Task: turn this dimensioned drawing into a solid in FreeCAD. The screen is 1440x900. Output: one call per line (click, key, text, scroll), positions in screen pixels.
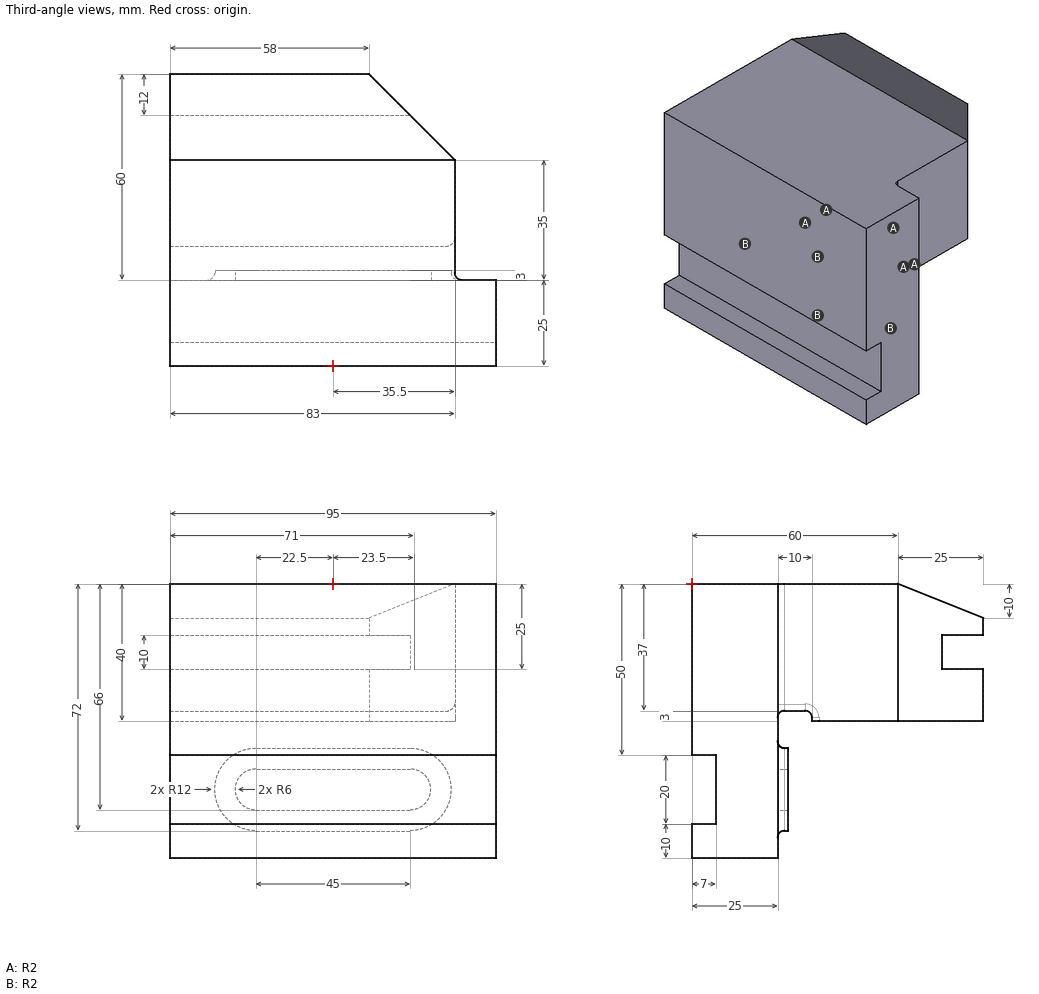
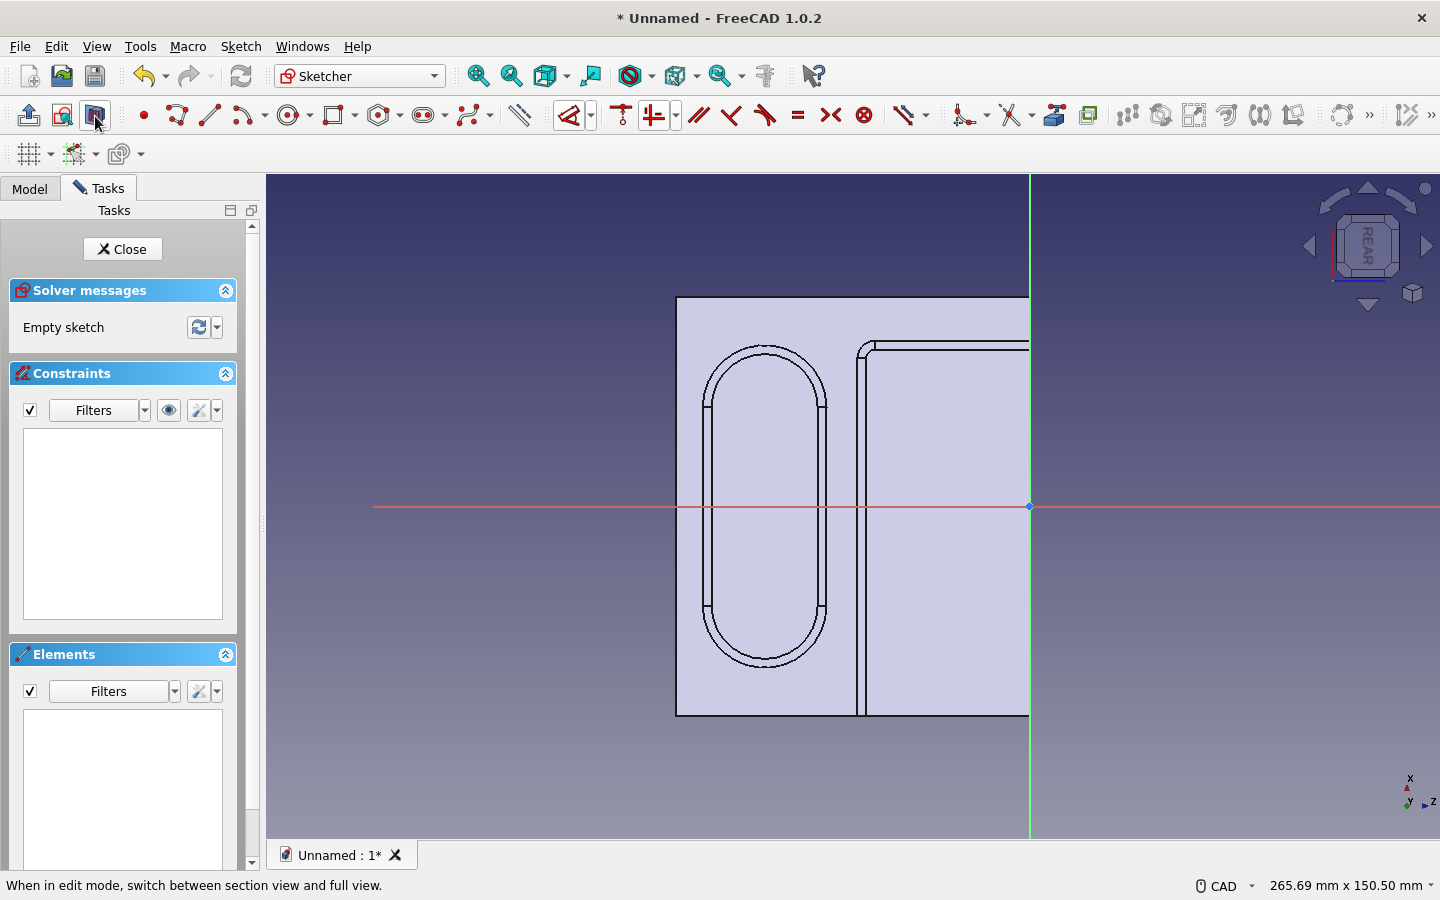
scroll(1005, 507, up, 3)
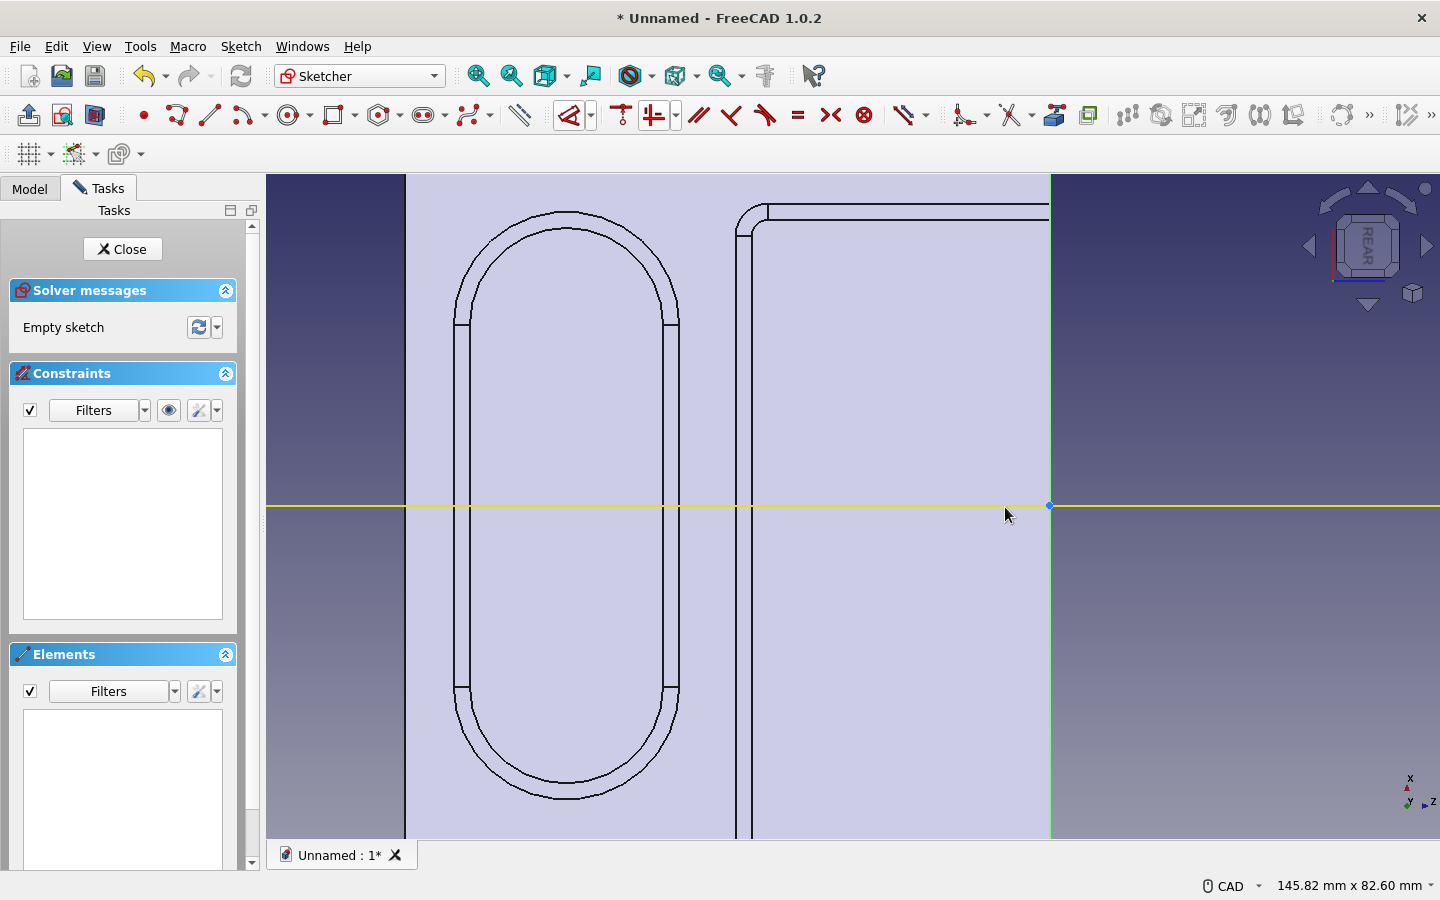
click(422, 116)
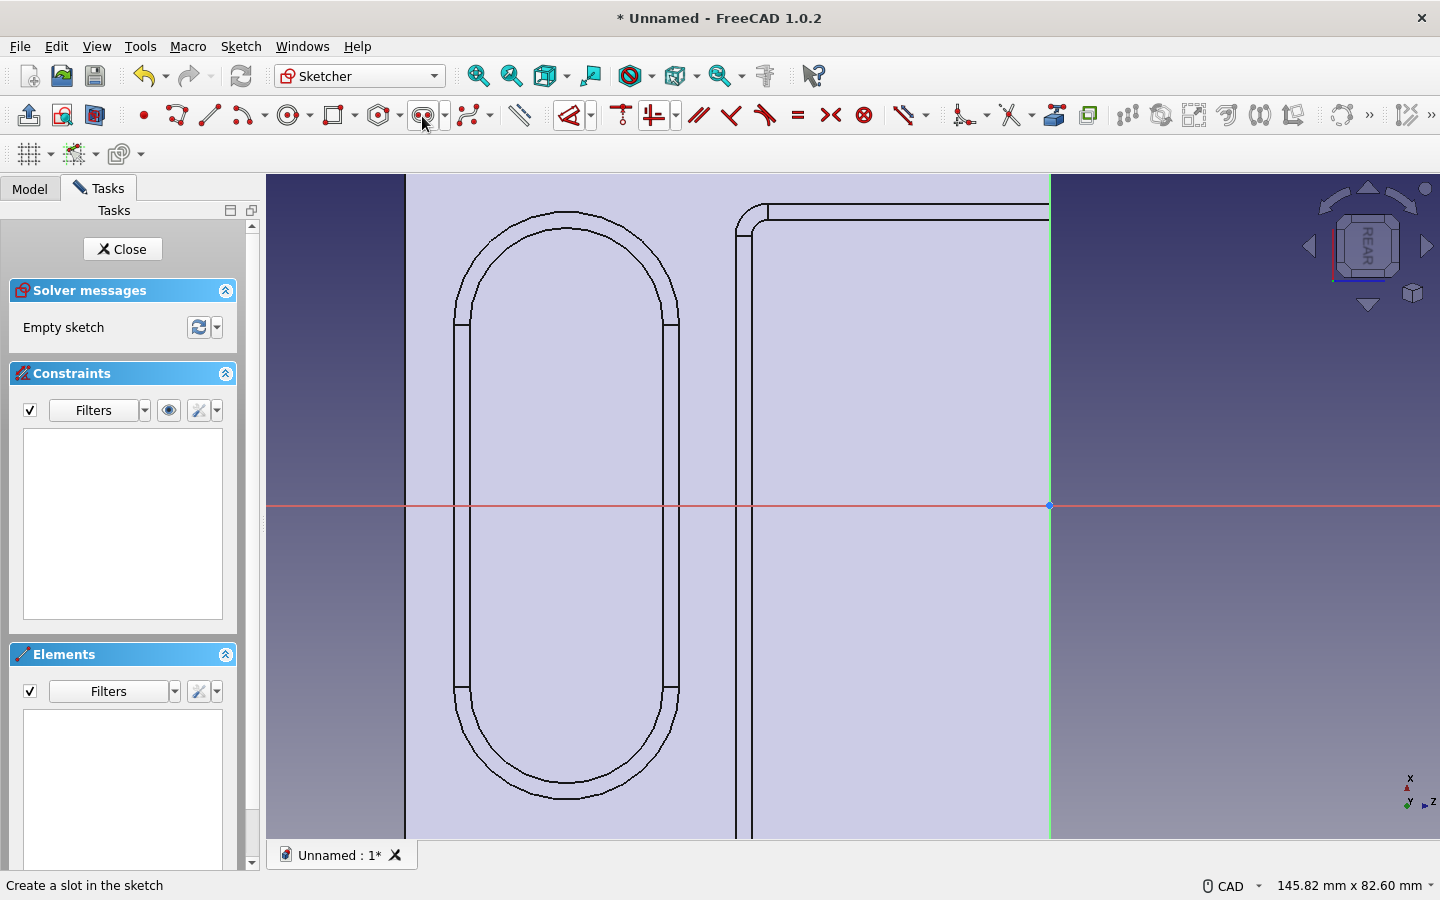
click(566, 687)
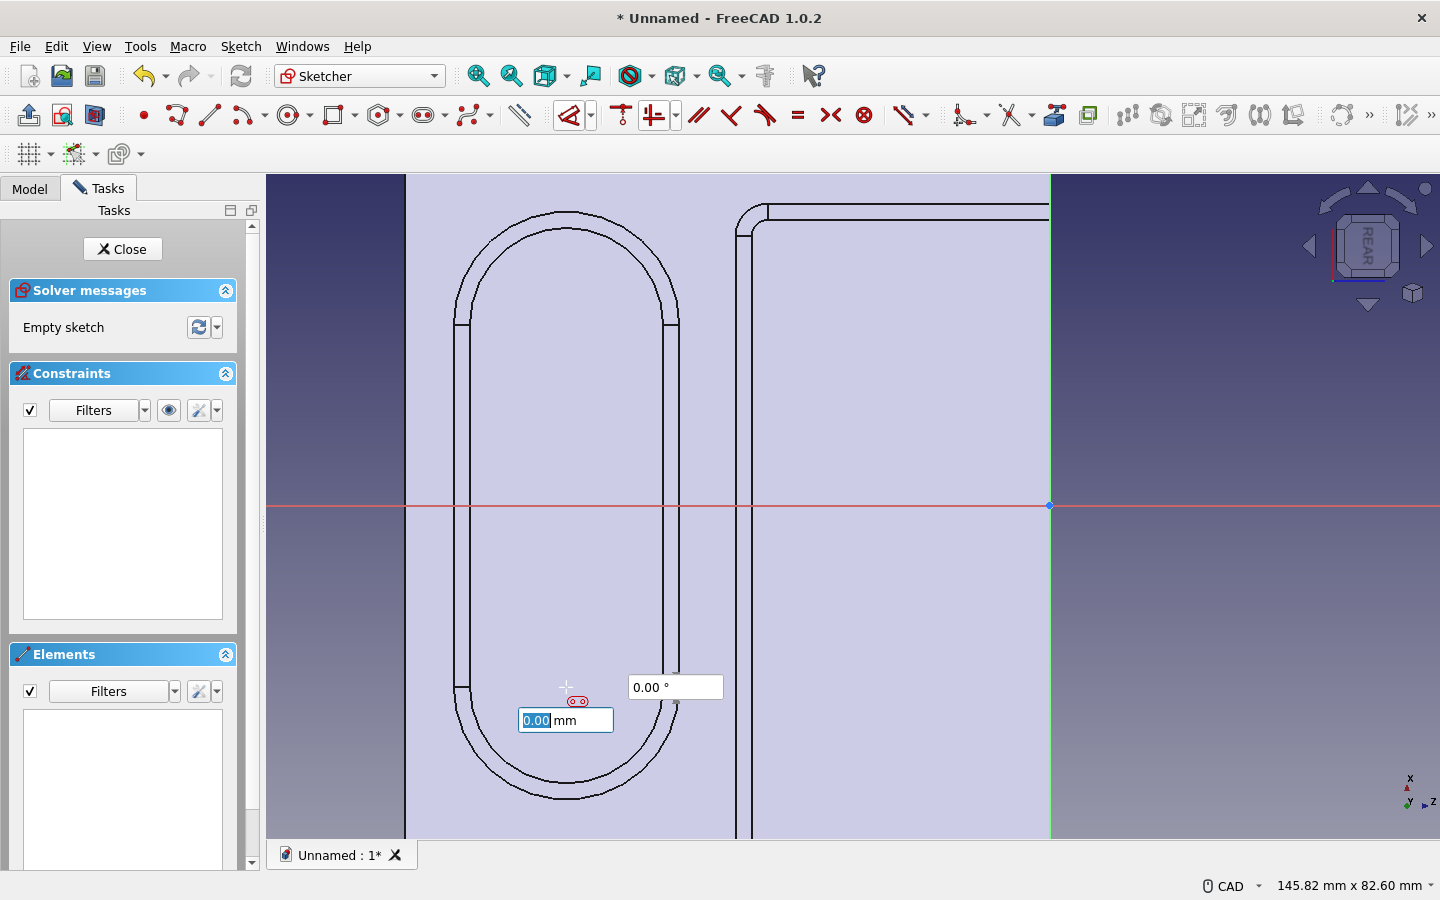
click(566, 325)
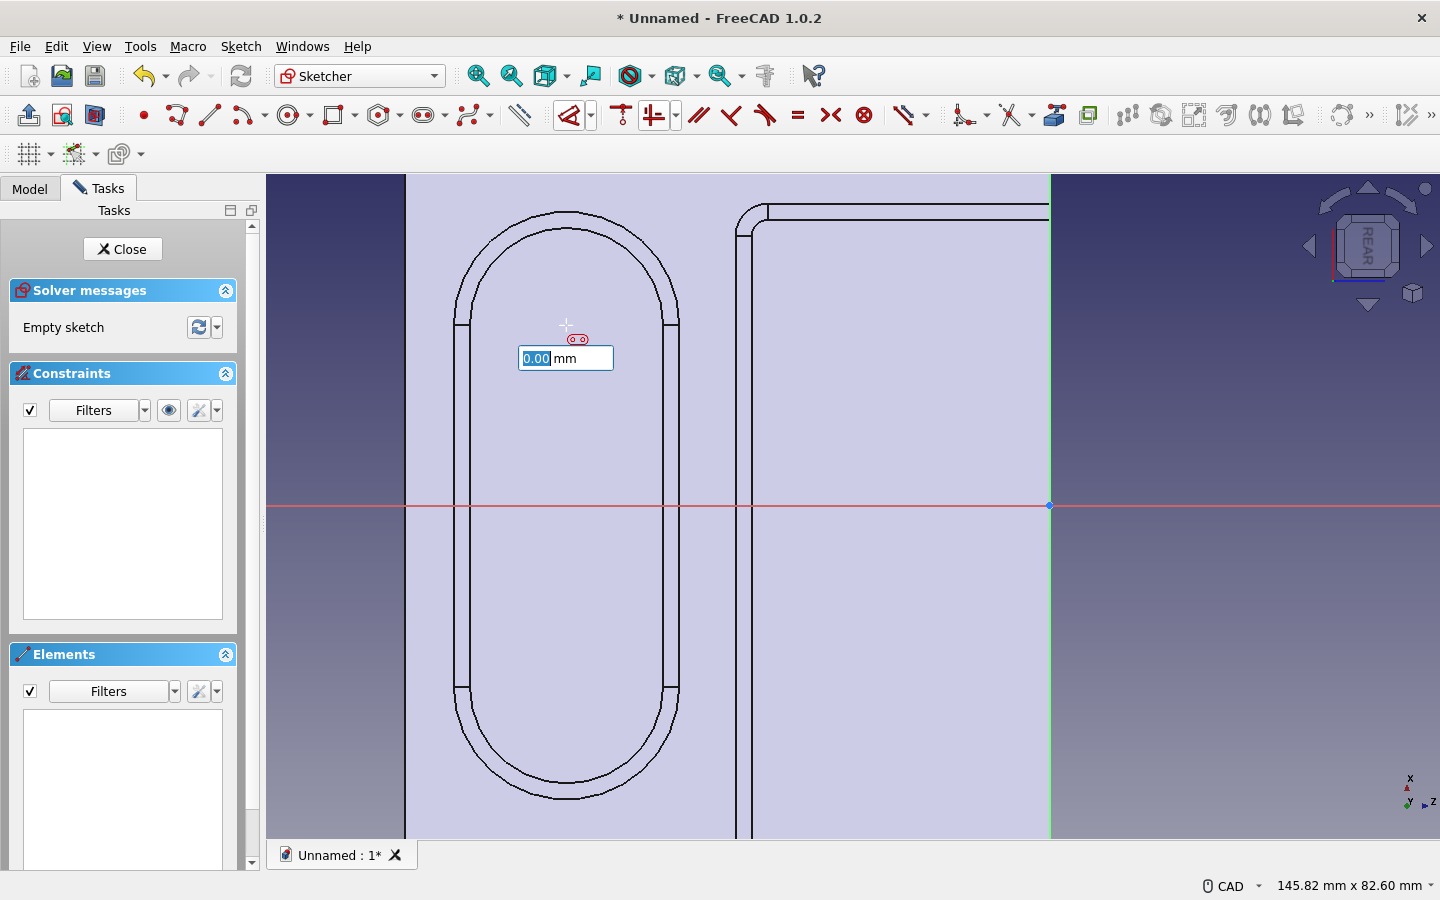
click(518, 451)
key(Escape)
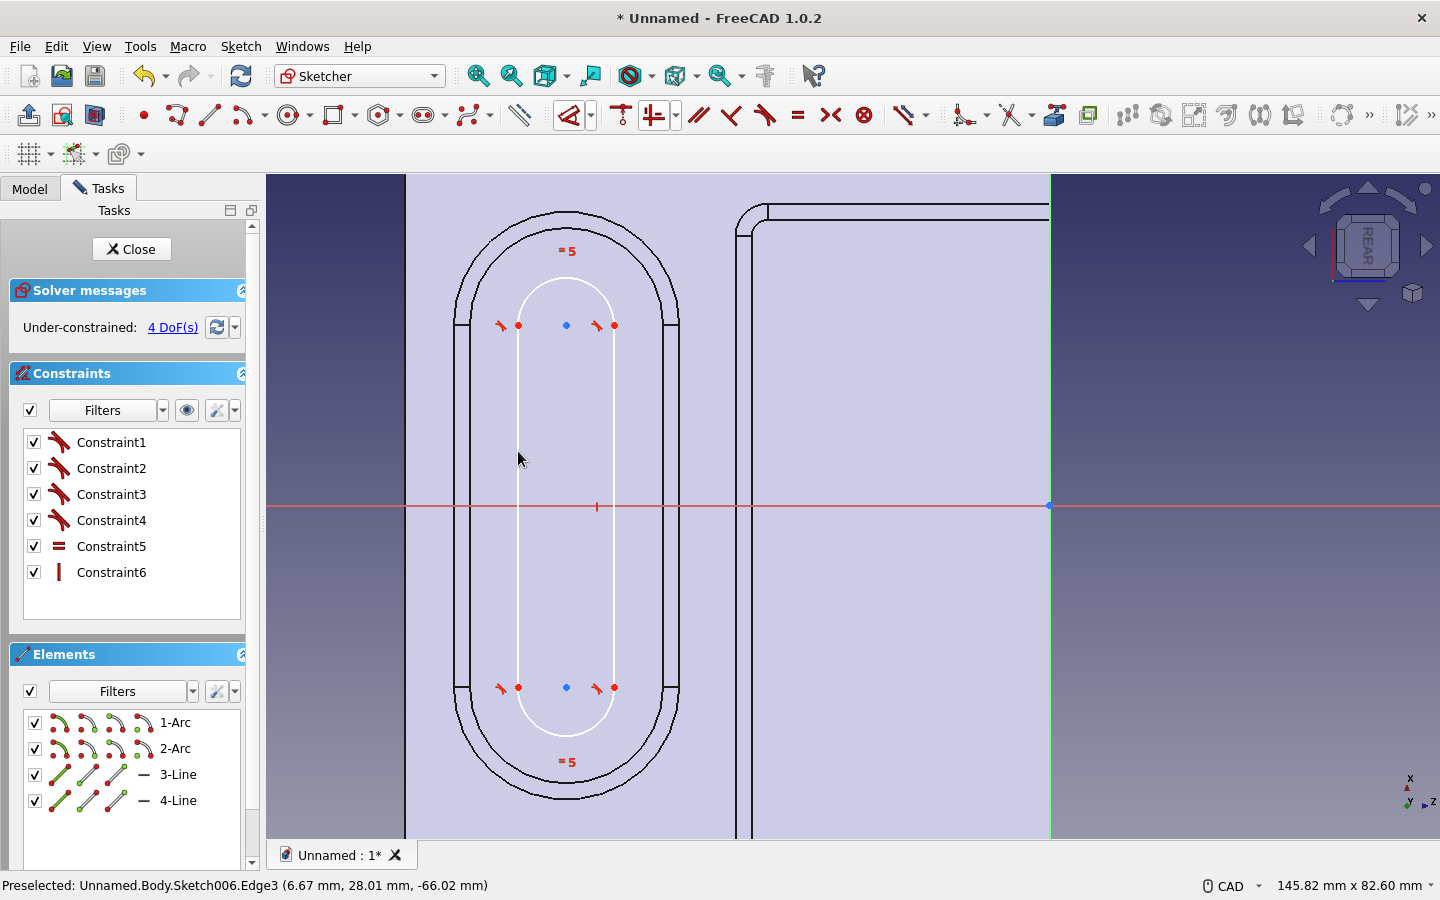
click(538, 727)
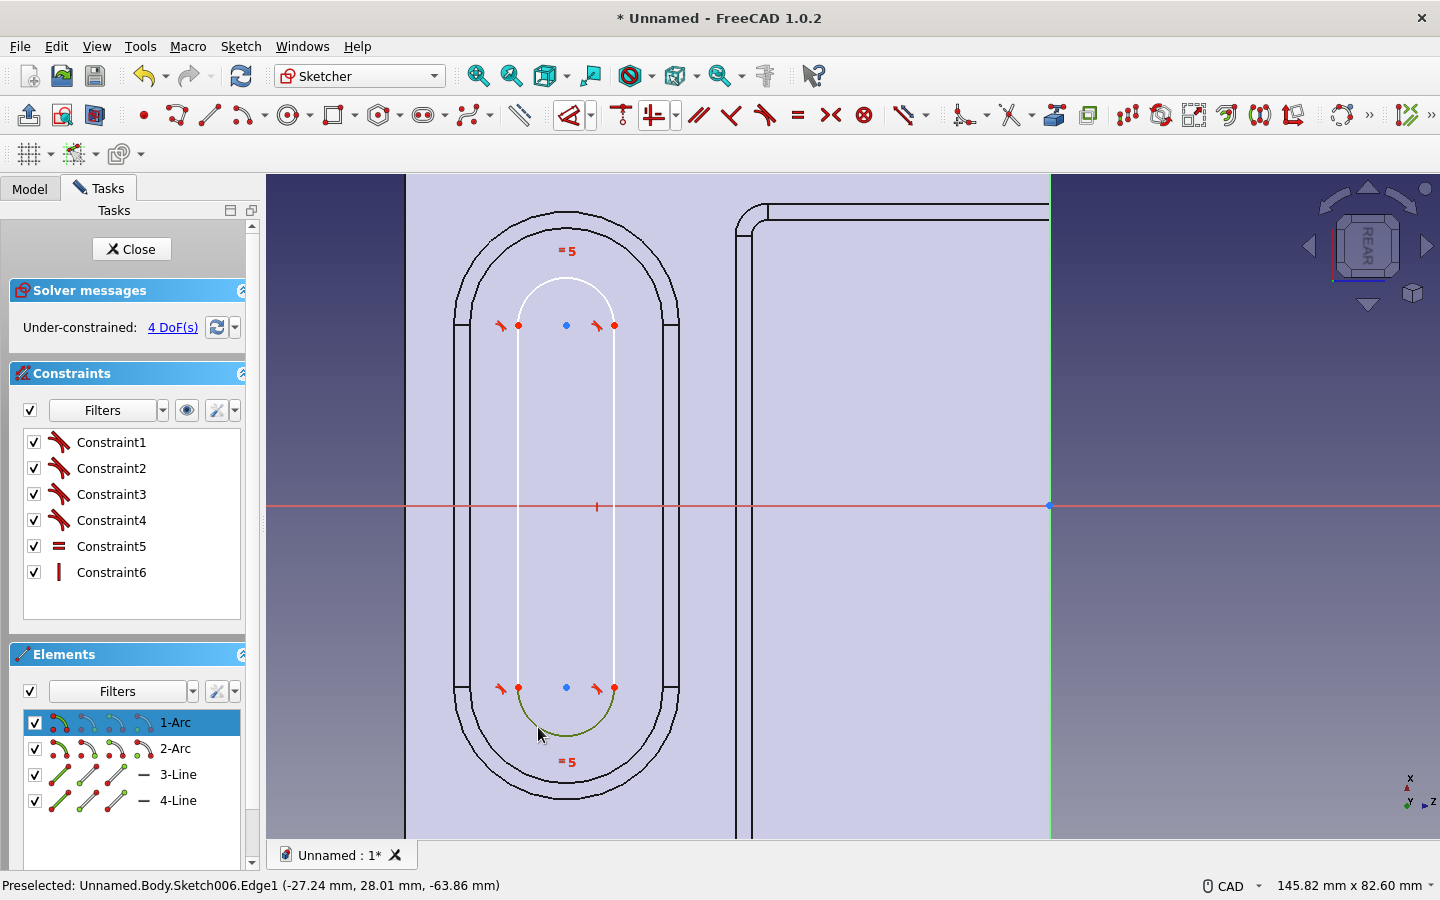
key(k)
key(r)